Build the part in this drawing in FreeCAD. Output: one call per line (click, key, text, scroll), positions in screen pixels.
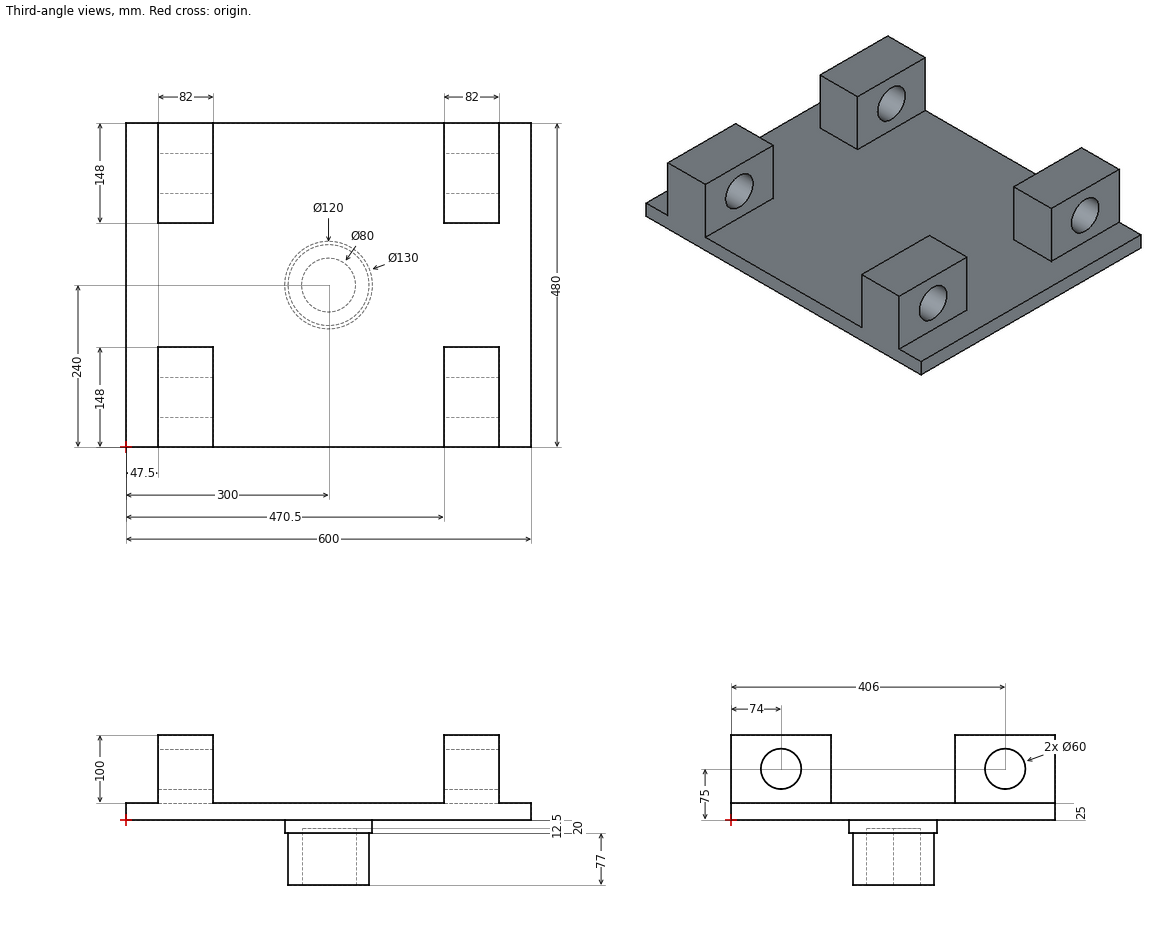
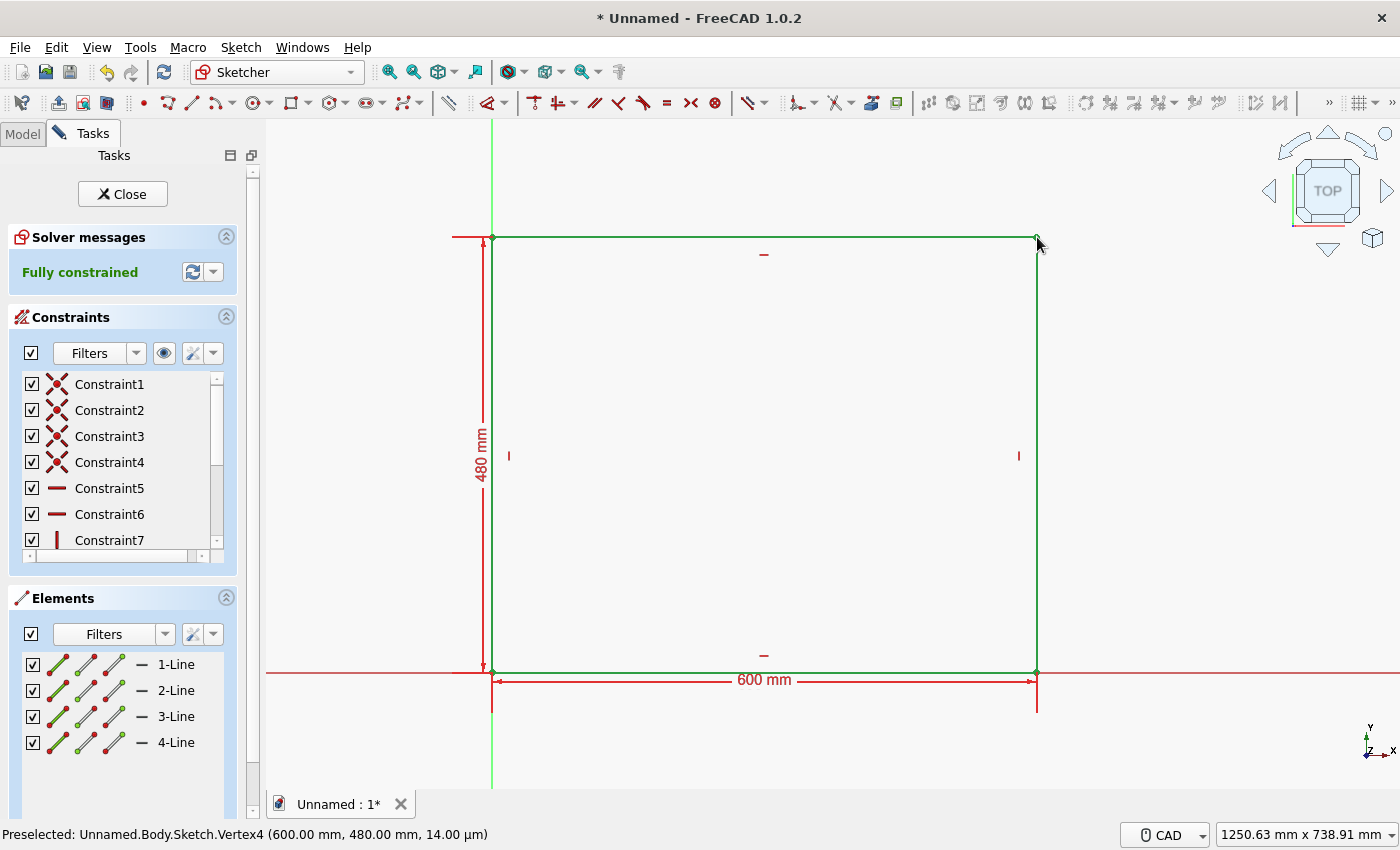
click(123, 194)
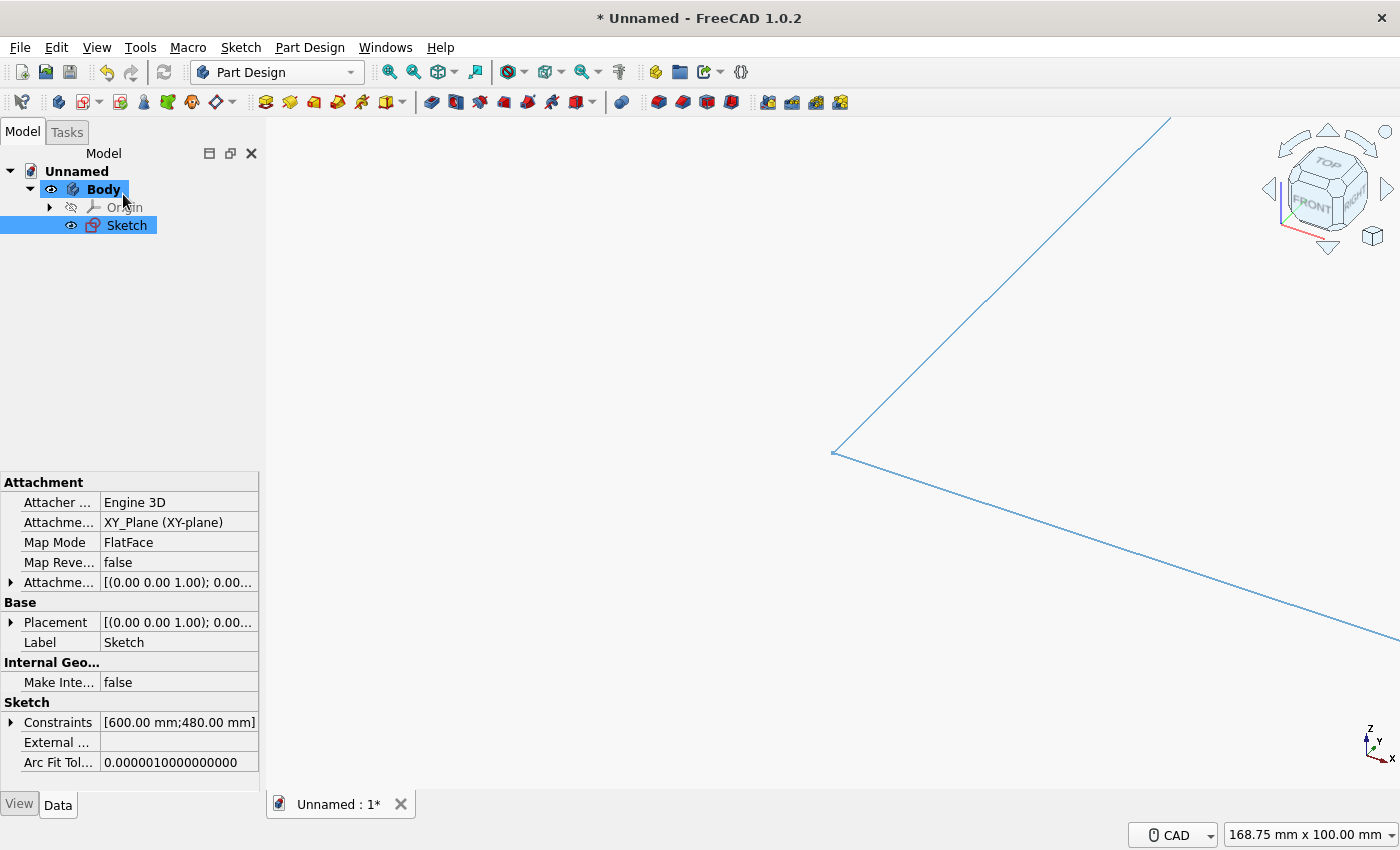
click(266, 102)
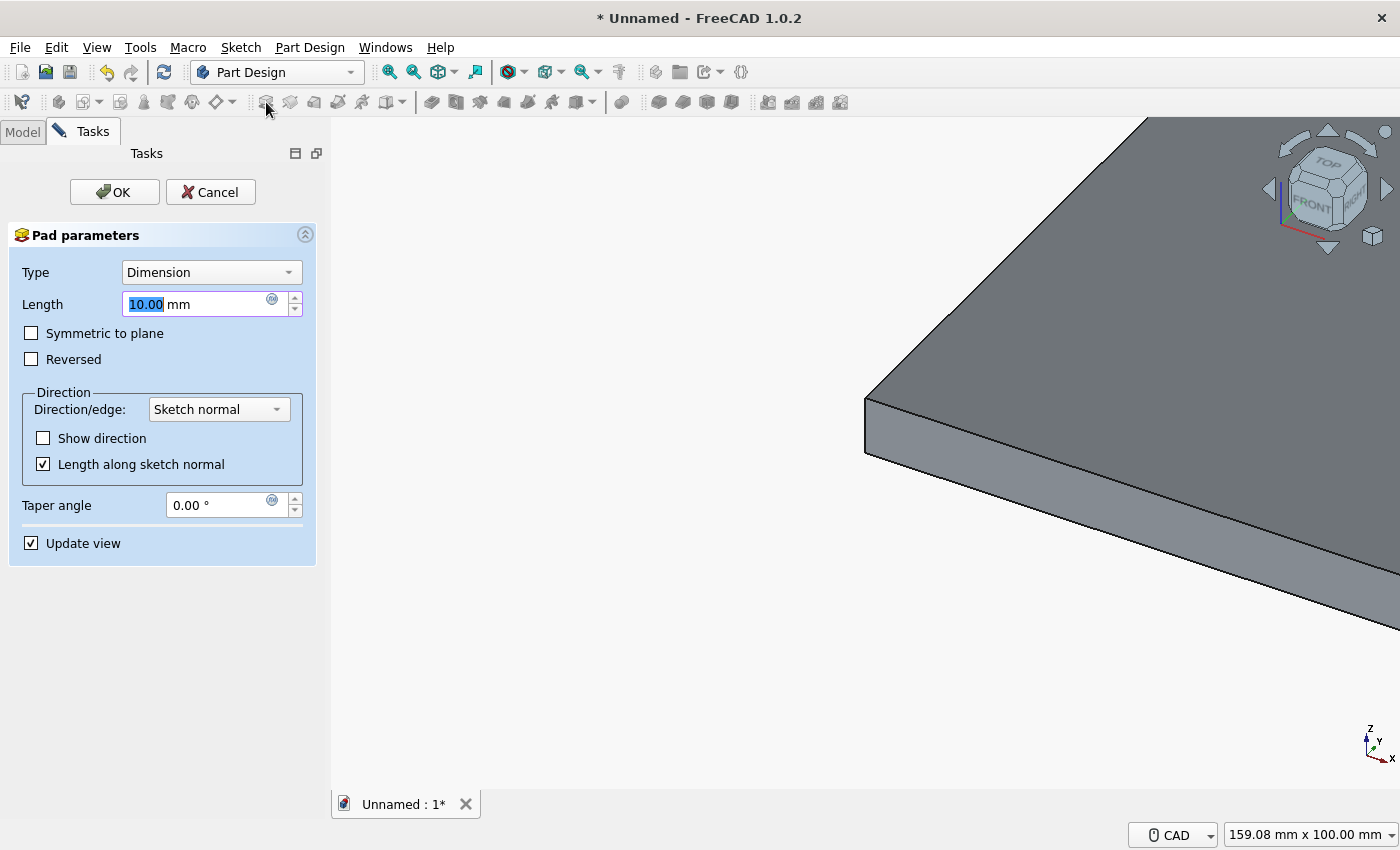
text(25)
key(Tab)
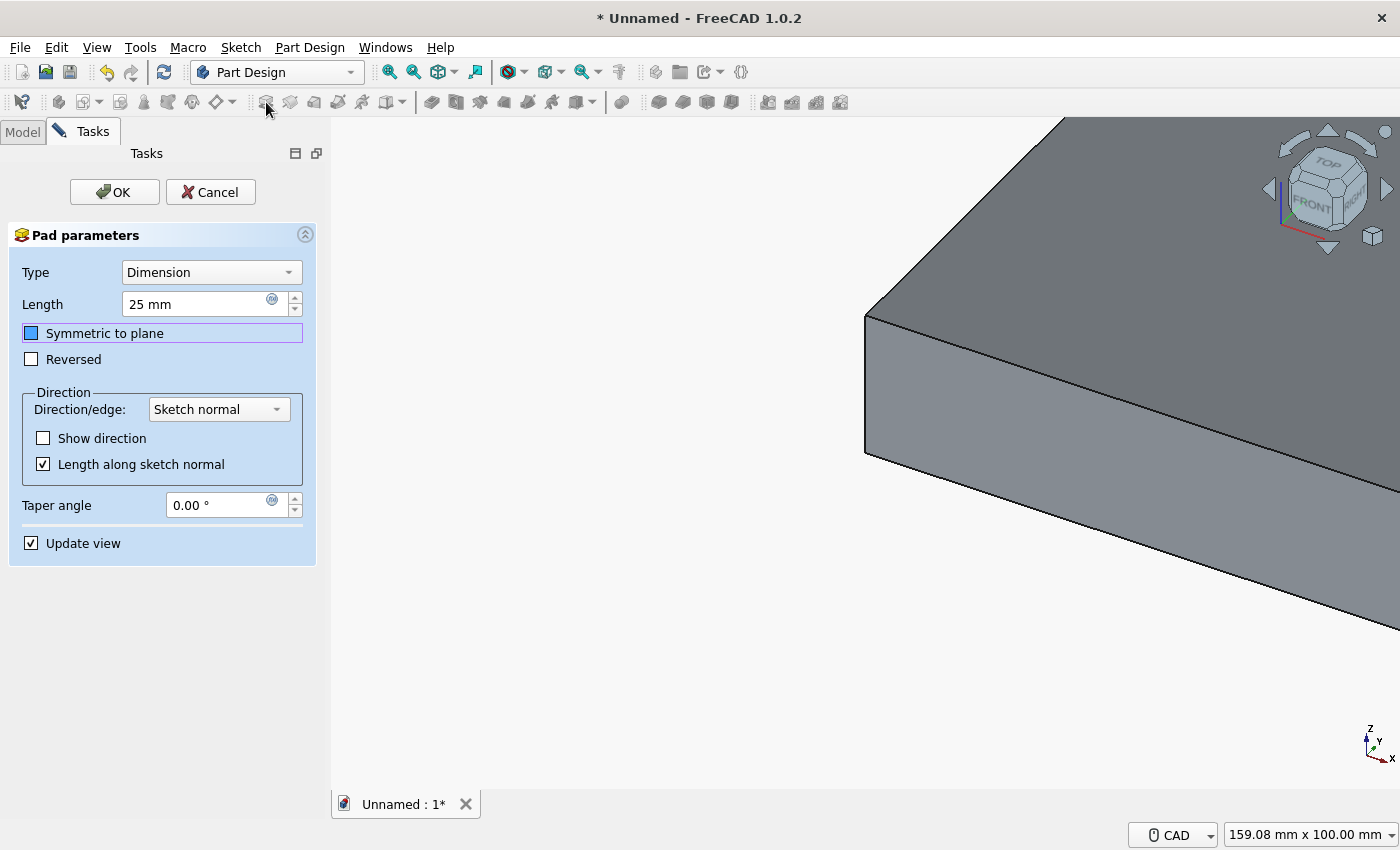
click(115, 192)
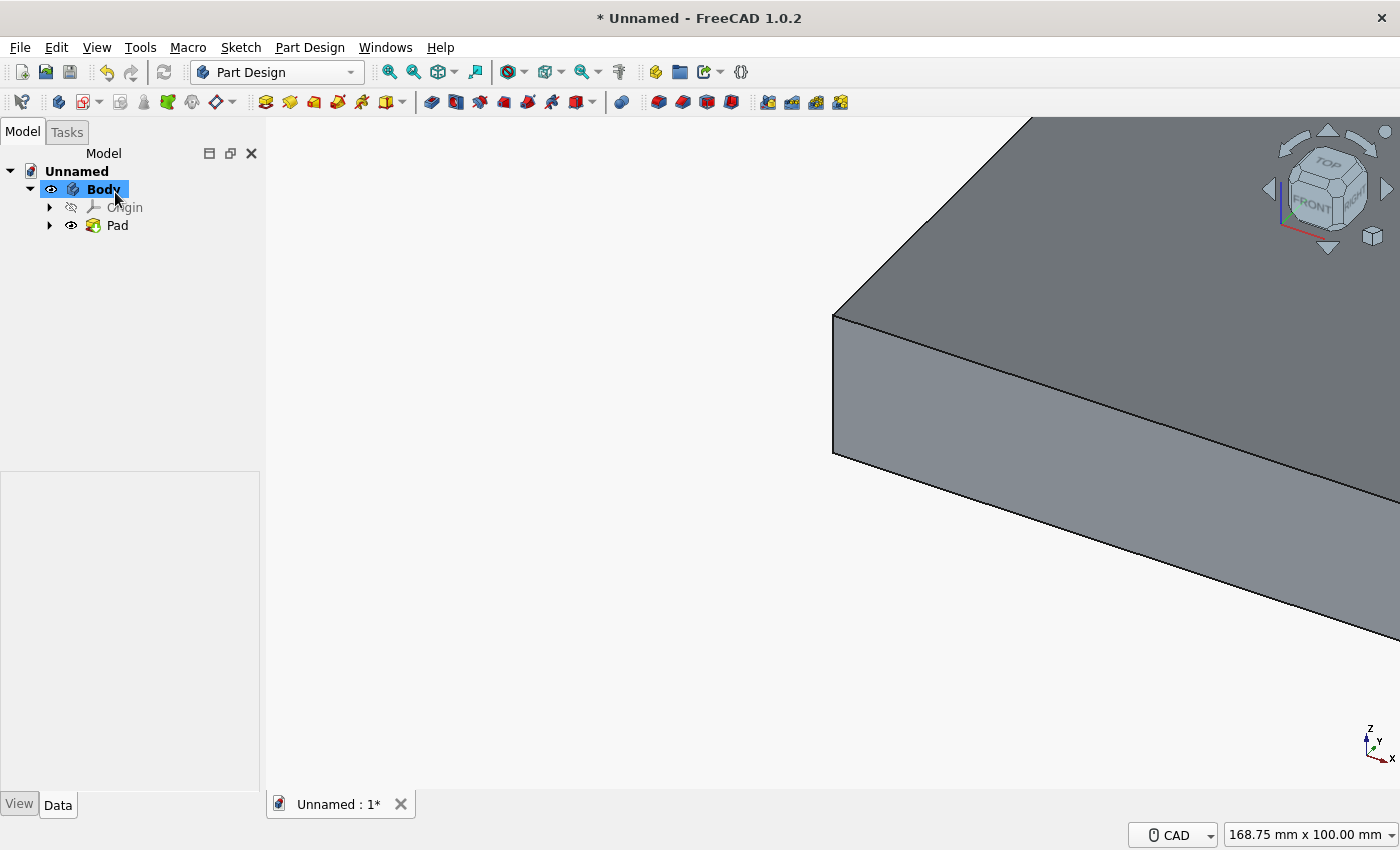
click(390, 72)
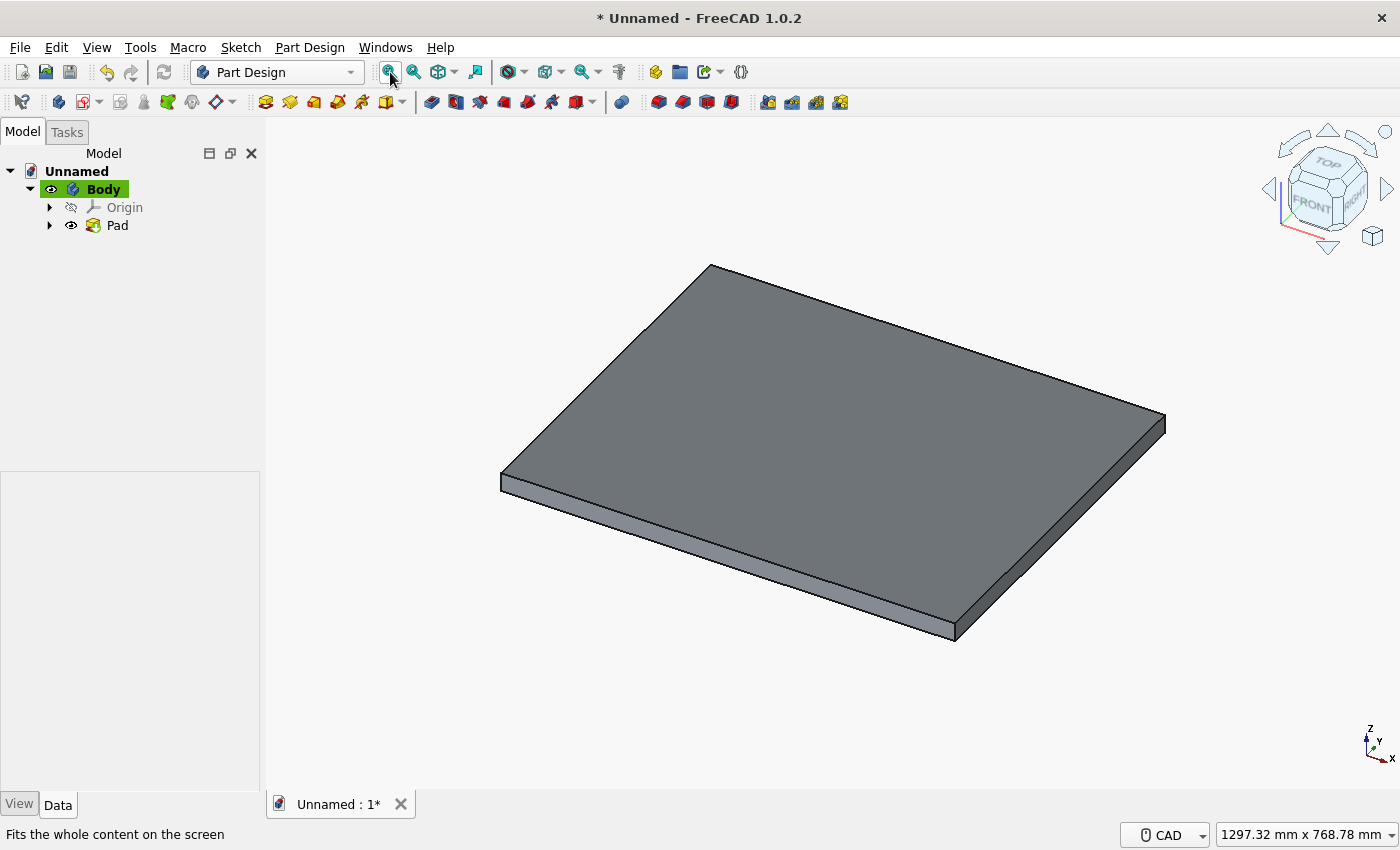
click(833, 443)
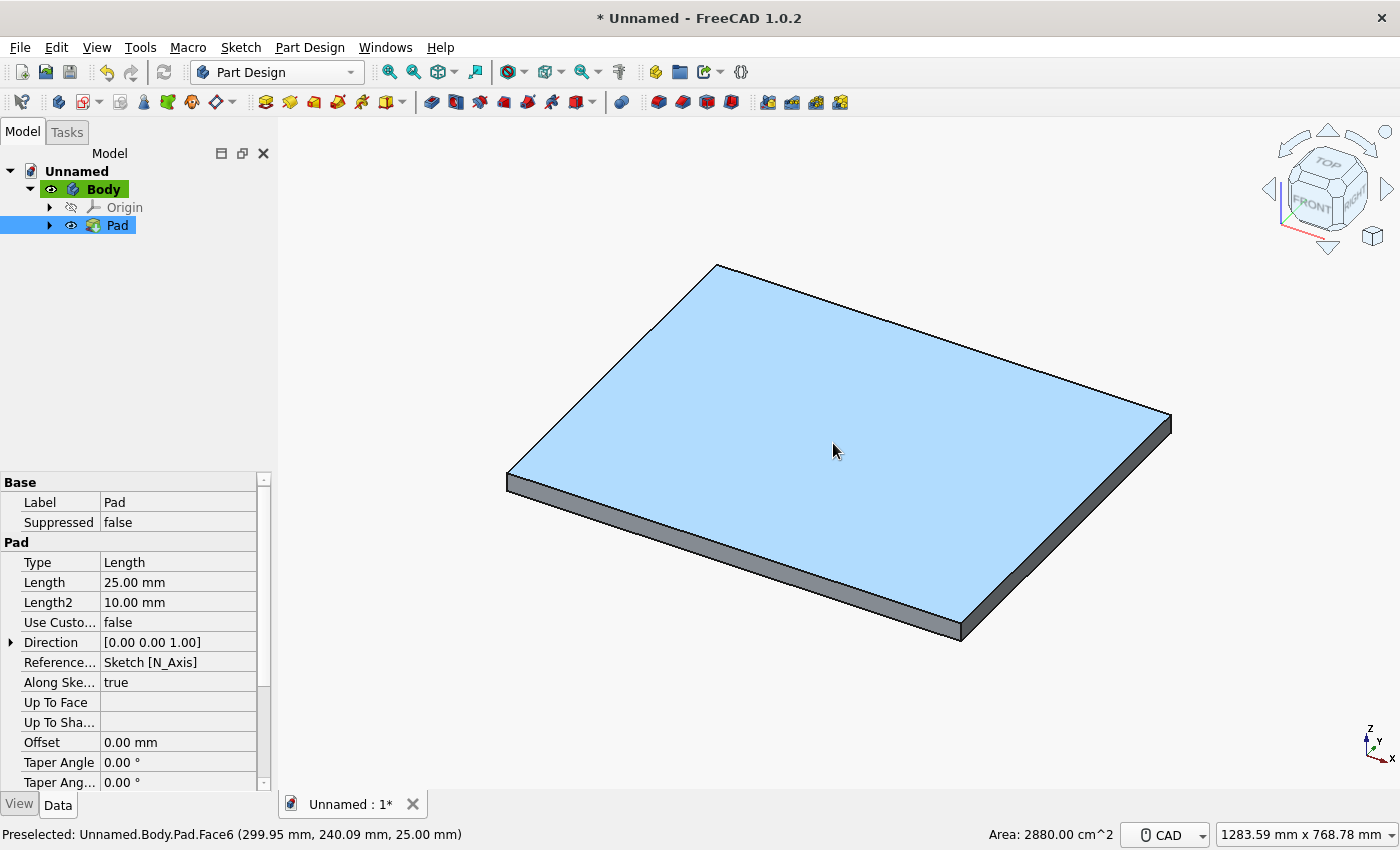
click(84, 102)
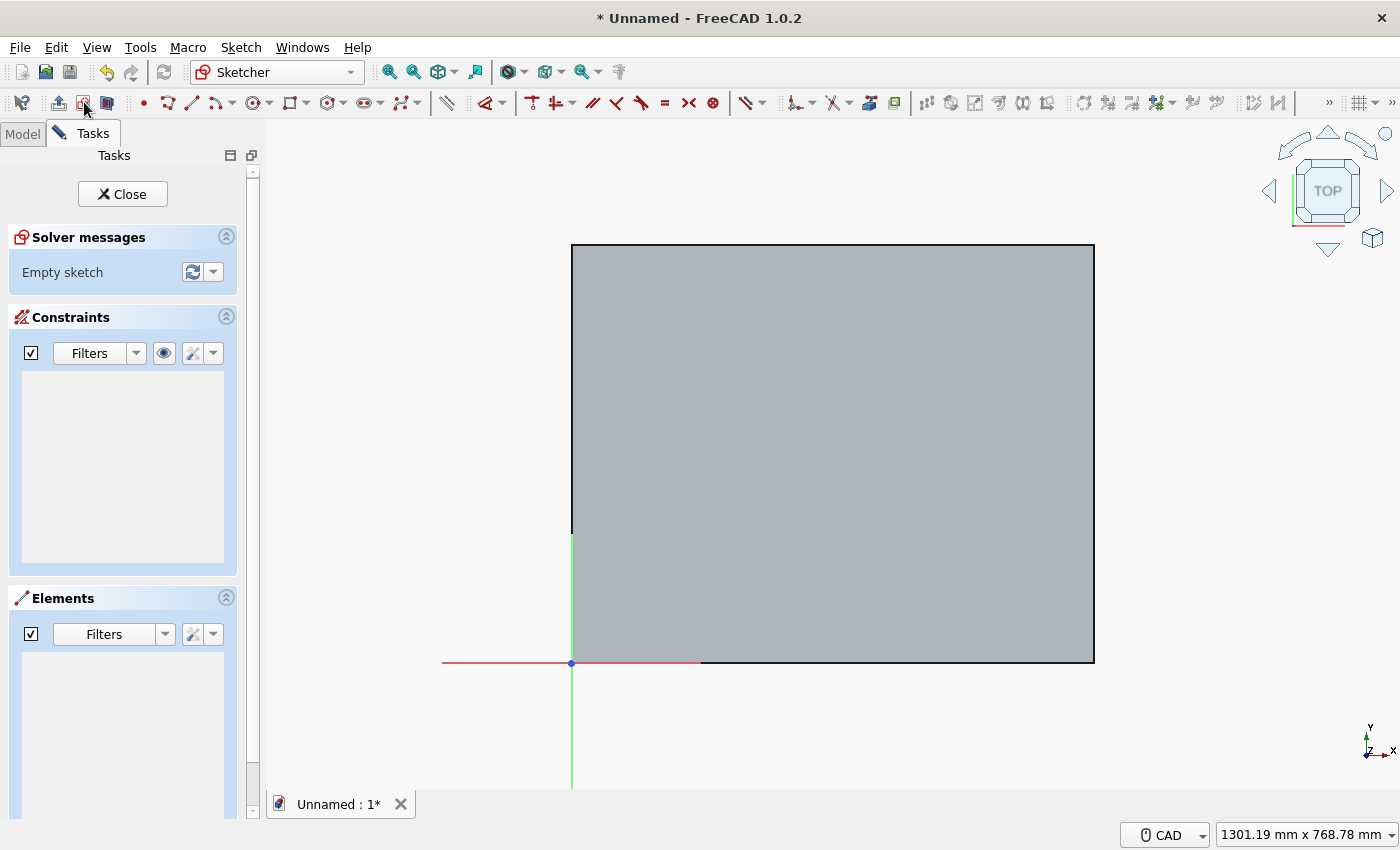
click(290, 104)